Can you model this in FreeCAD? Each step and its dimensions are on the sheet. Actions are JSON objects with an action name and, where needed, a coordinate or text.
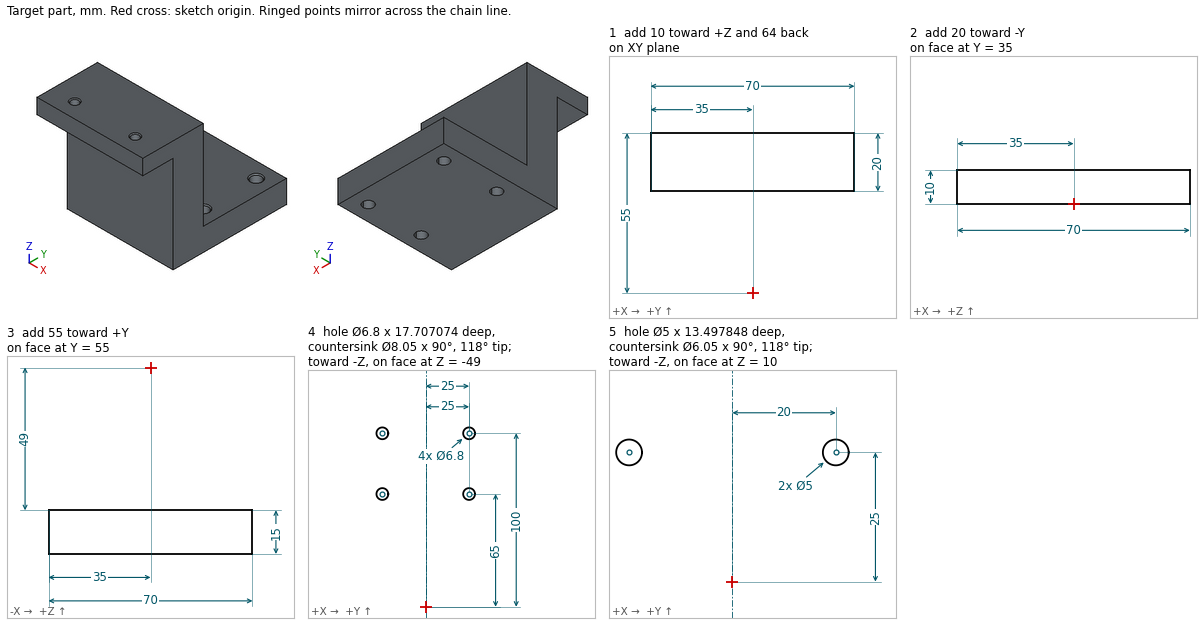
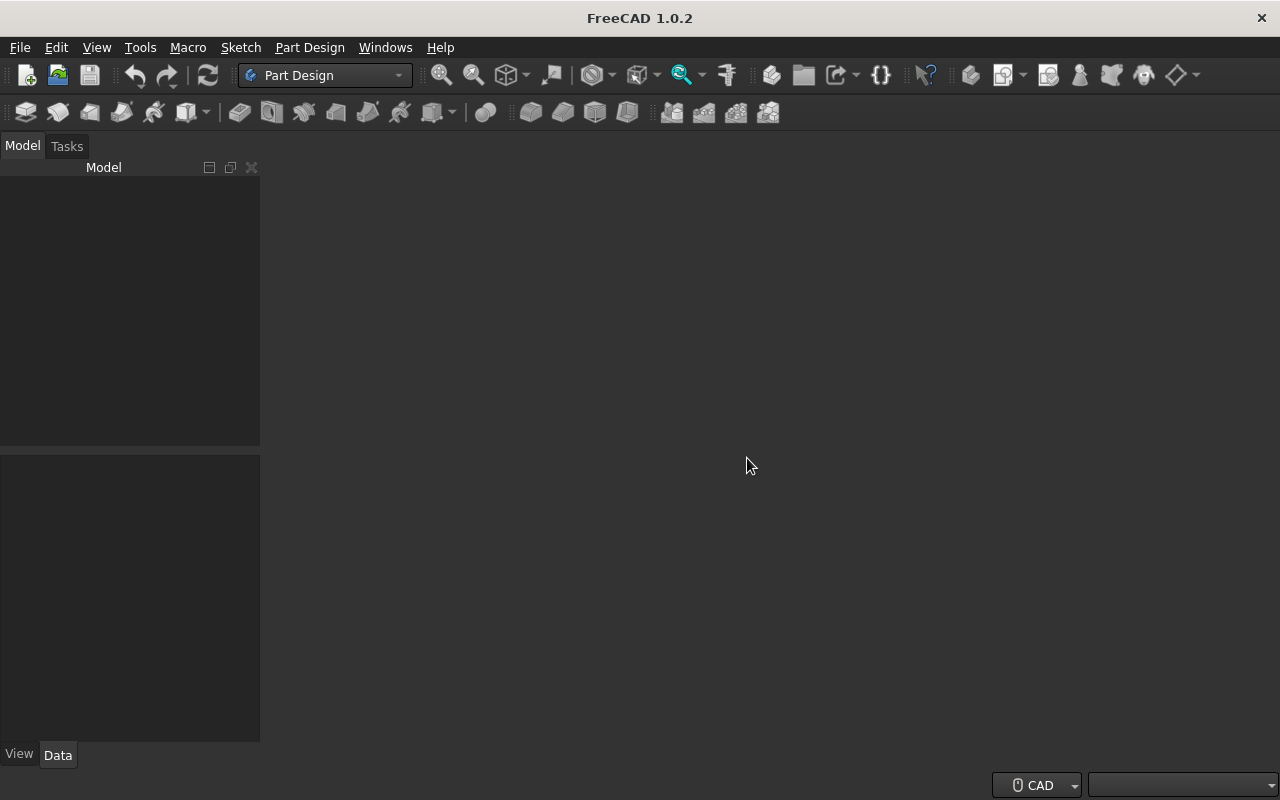
{"action": "left_click", "coordinate": [26, 76]}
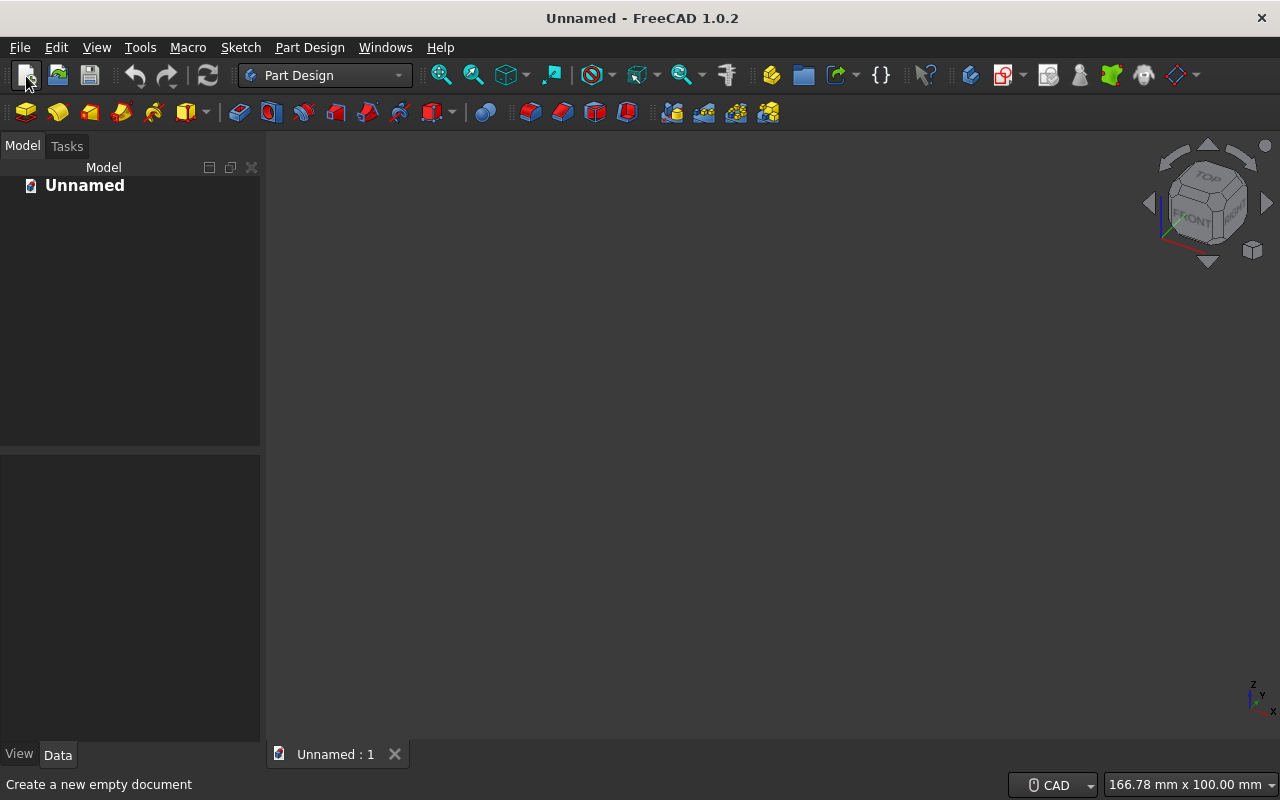
{"action": "left_click", "coordinate": [1004, 76]}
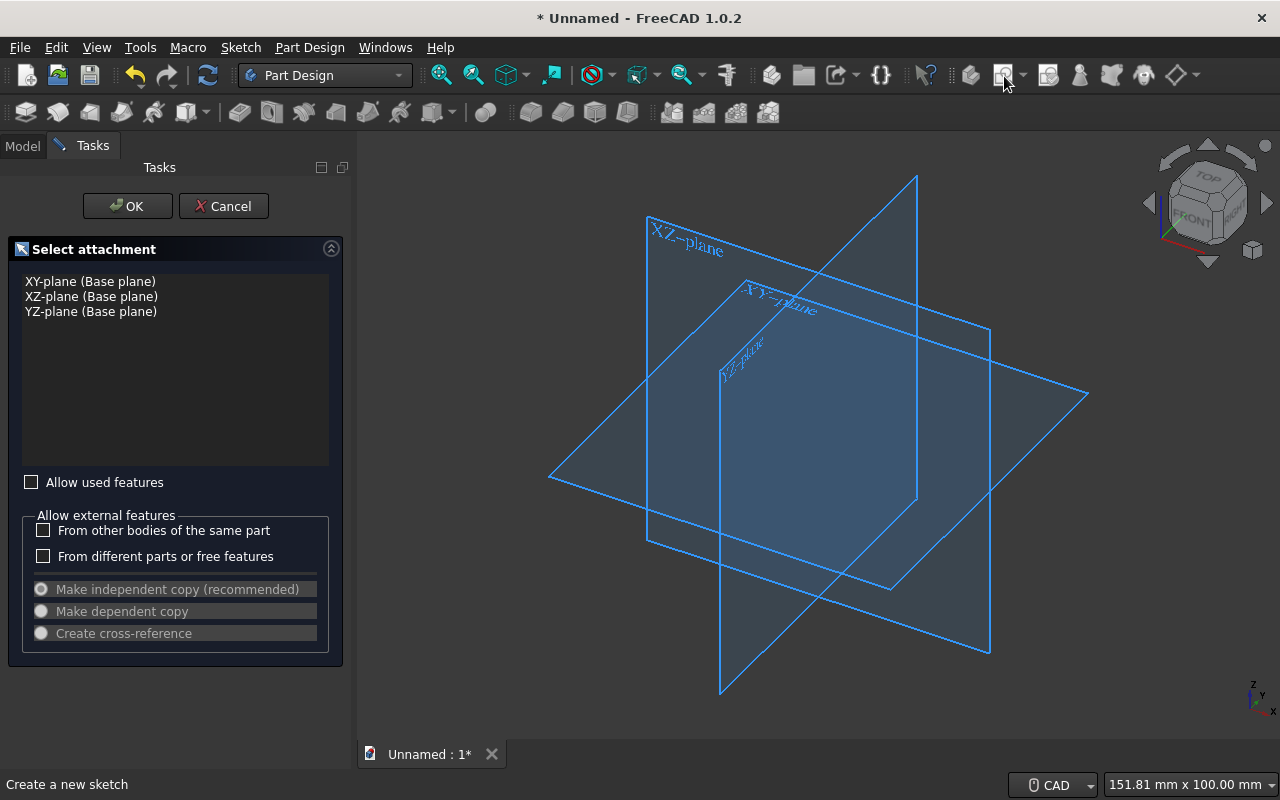
{"action": "left_click", "coordinate": [82, 282]}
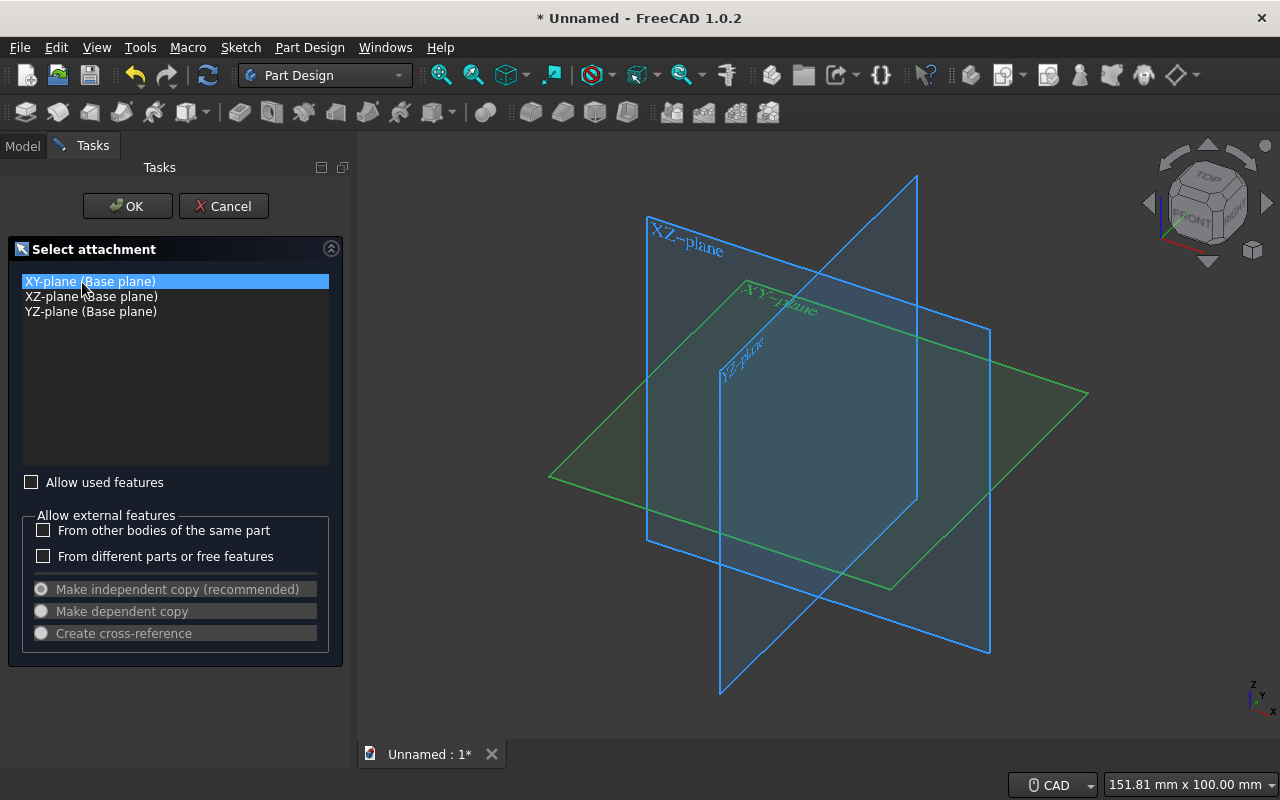
{"action": "left_click", "coordinate": [128, 206]}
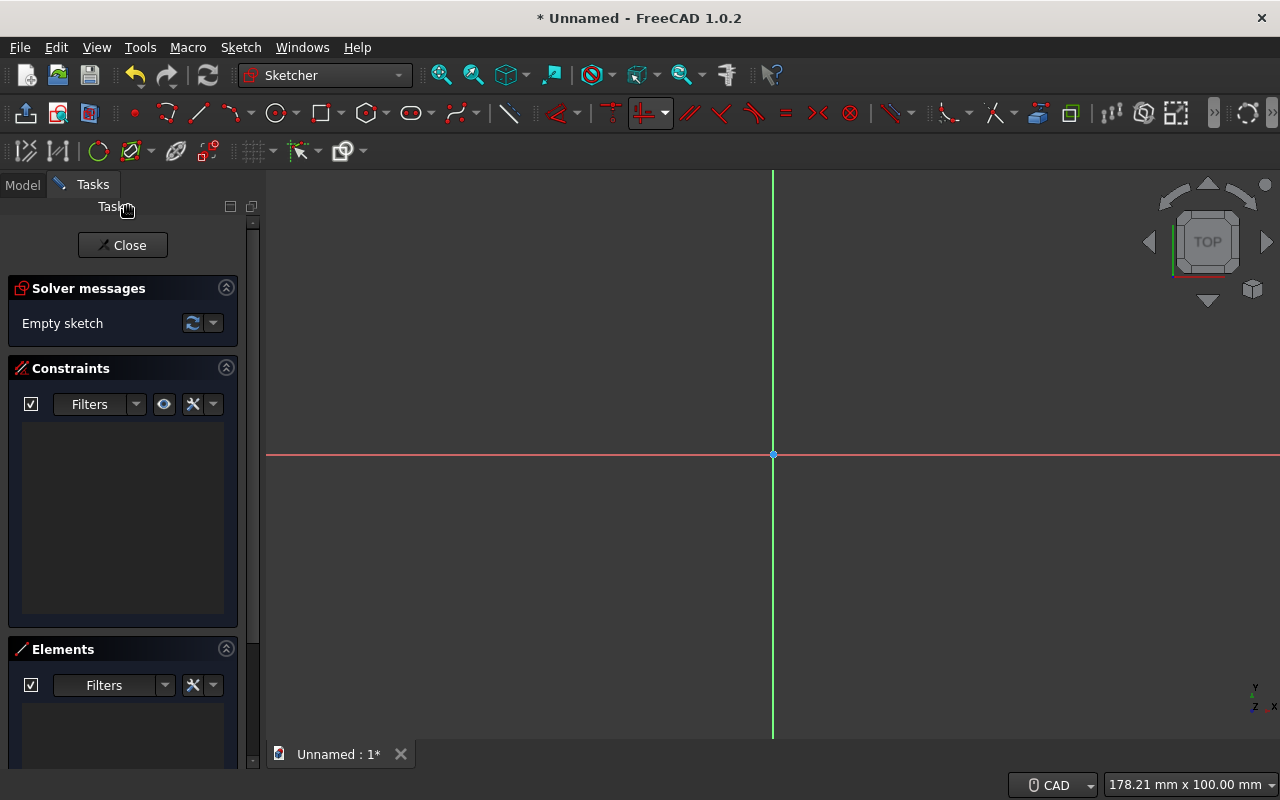
{"action": "scroll", "coordinate": [395, 711], "scroll_direction": "down", "scroll_amount": 1}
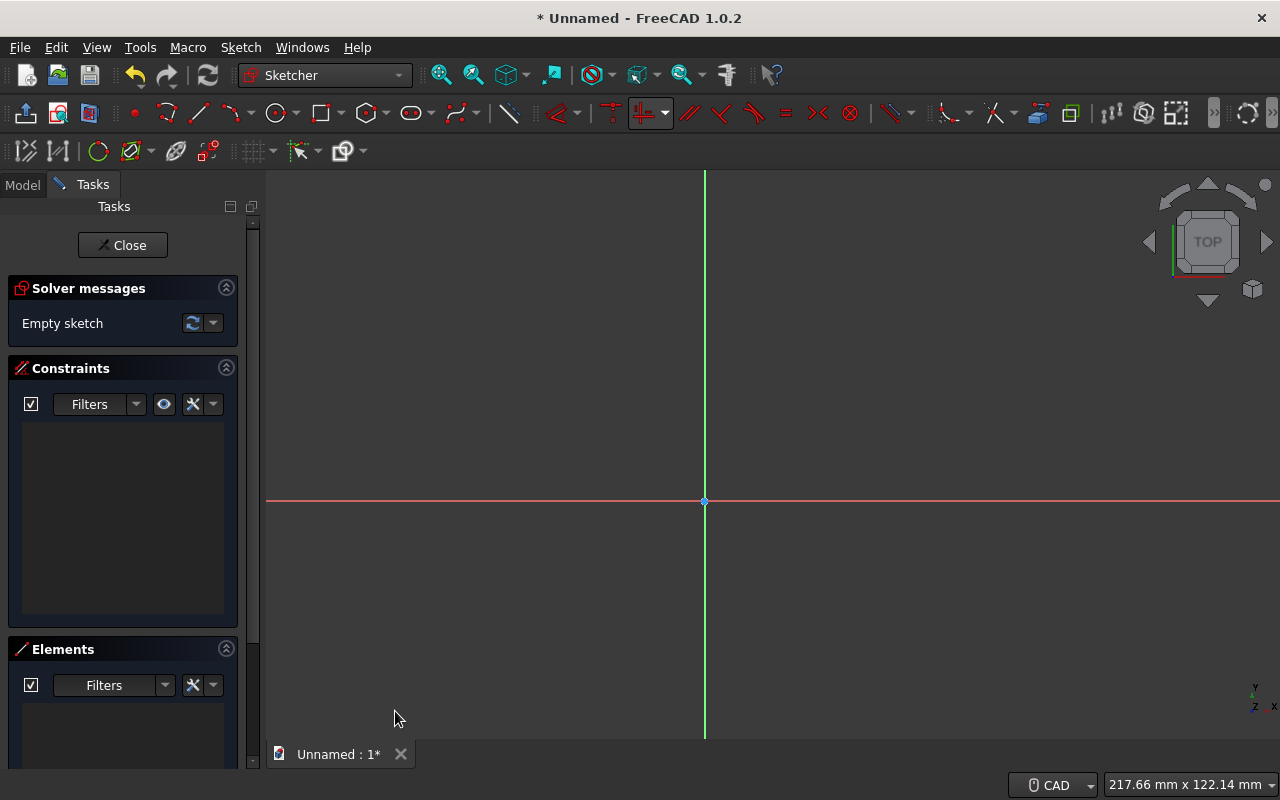
{"action": "scroll", "coordinate": [705, 207], "scroll_direction": "up", "scroll_amount": 2}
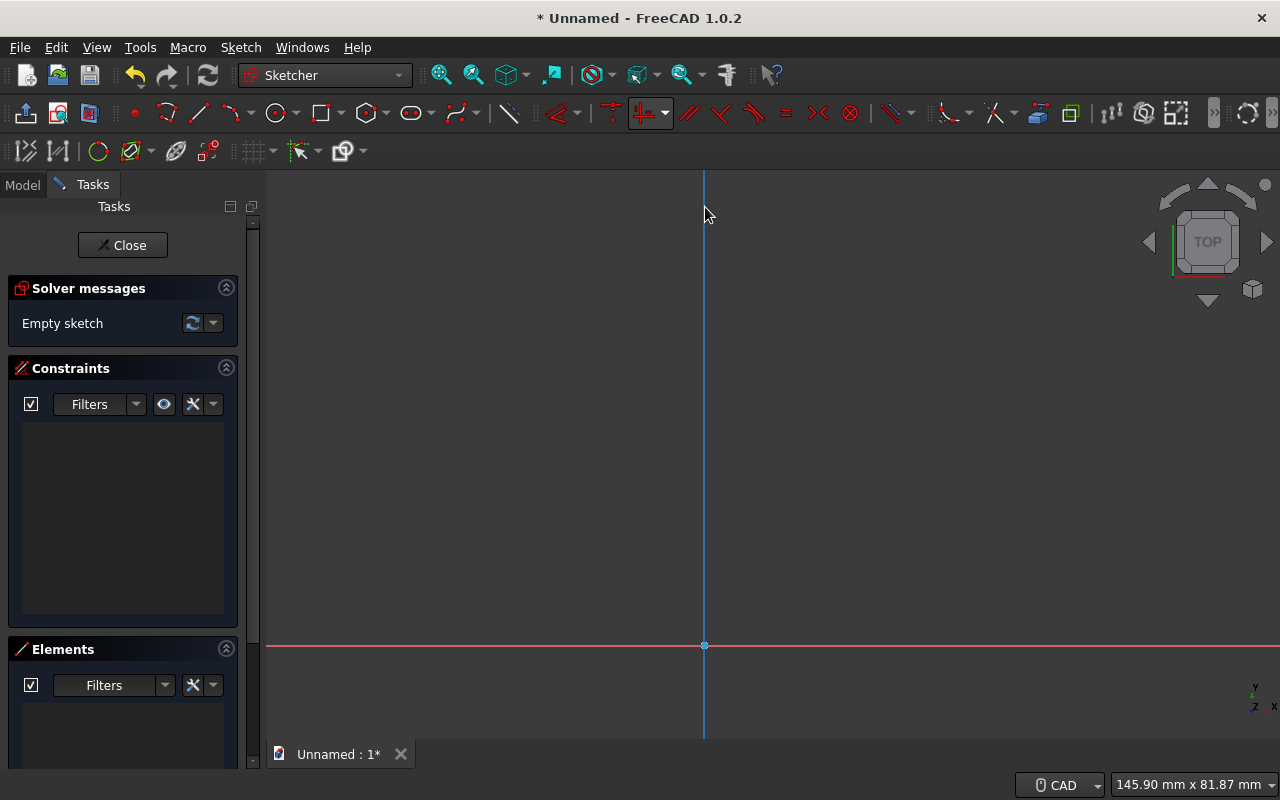
{"action": "key", "text": "g r"}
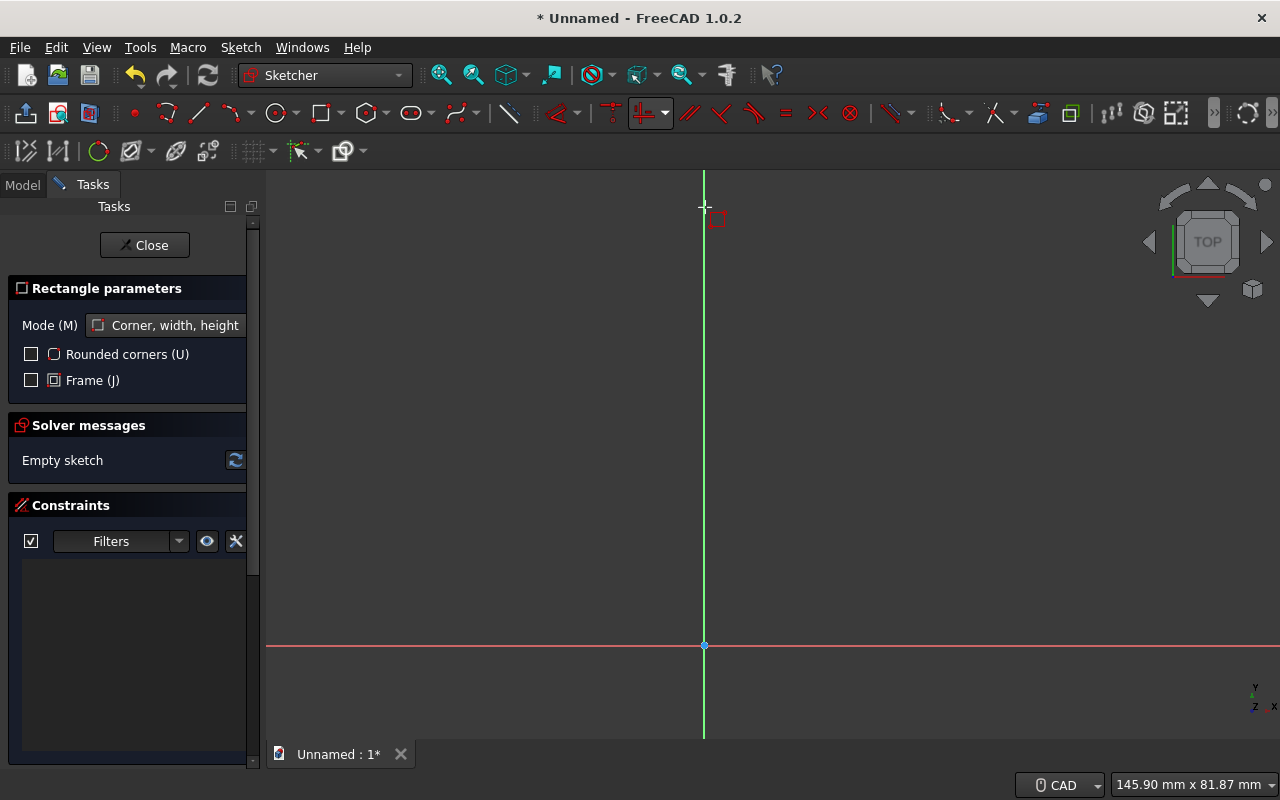
{"action": "left_click", "coordinate": [461, 264]}
{"action": "mouse_move", "coordinate": [947, 403]}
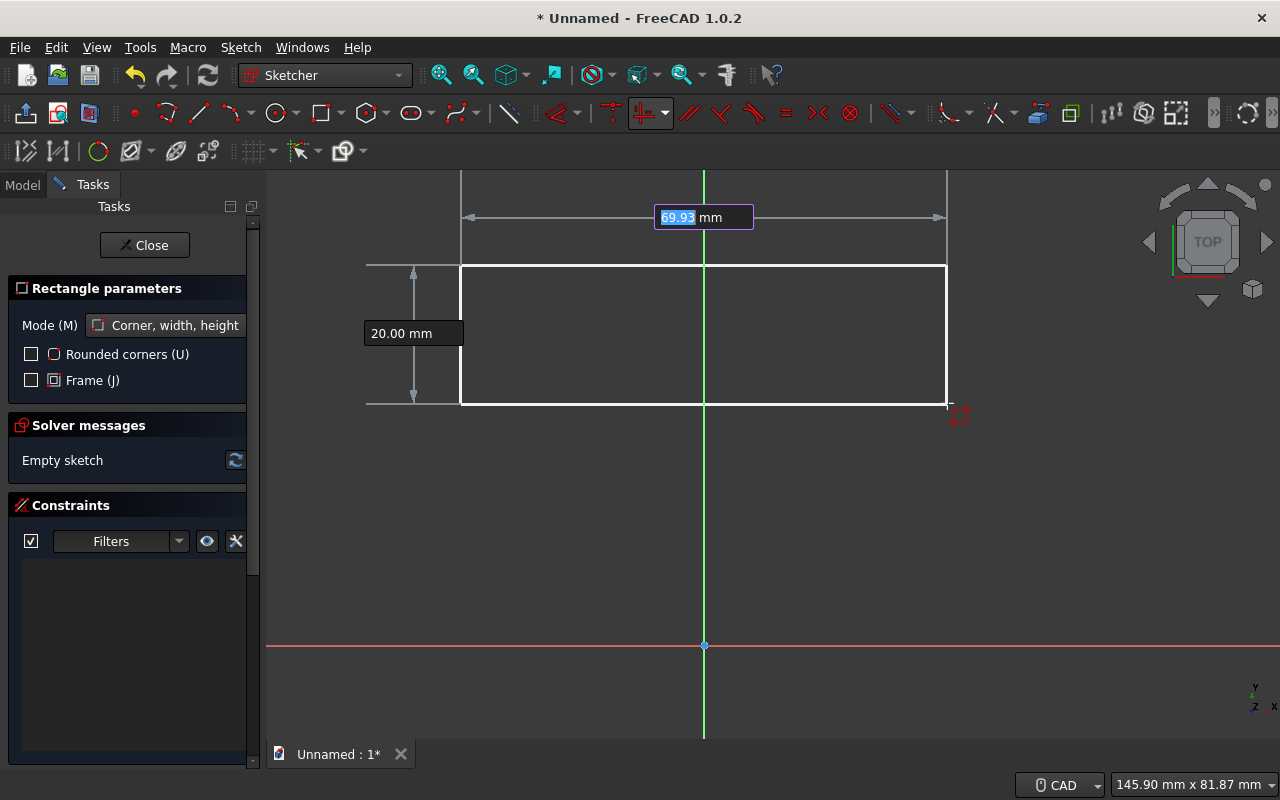
{"action": "type", "text": "70"}
{"action": "key", "text": "Tab"}
{"action": "type", "text": "20"}
{"action": "key", "text": "Return"}
{"action": "key", "text": "Escape"}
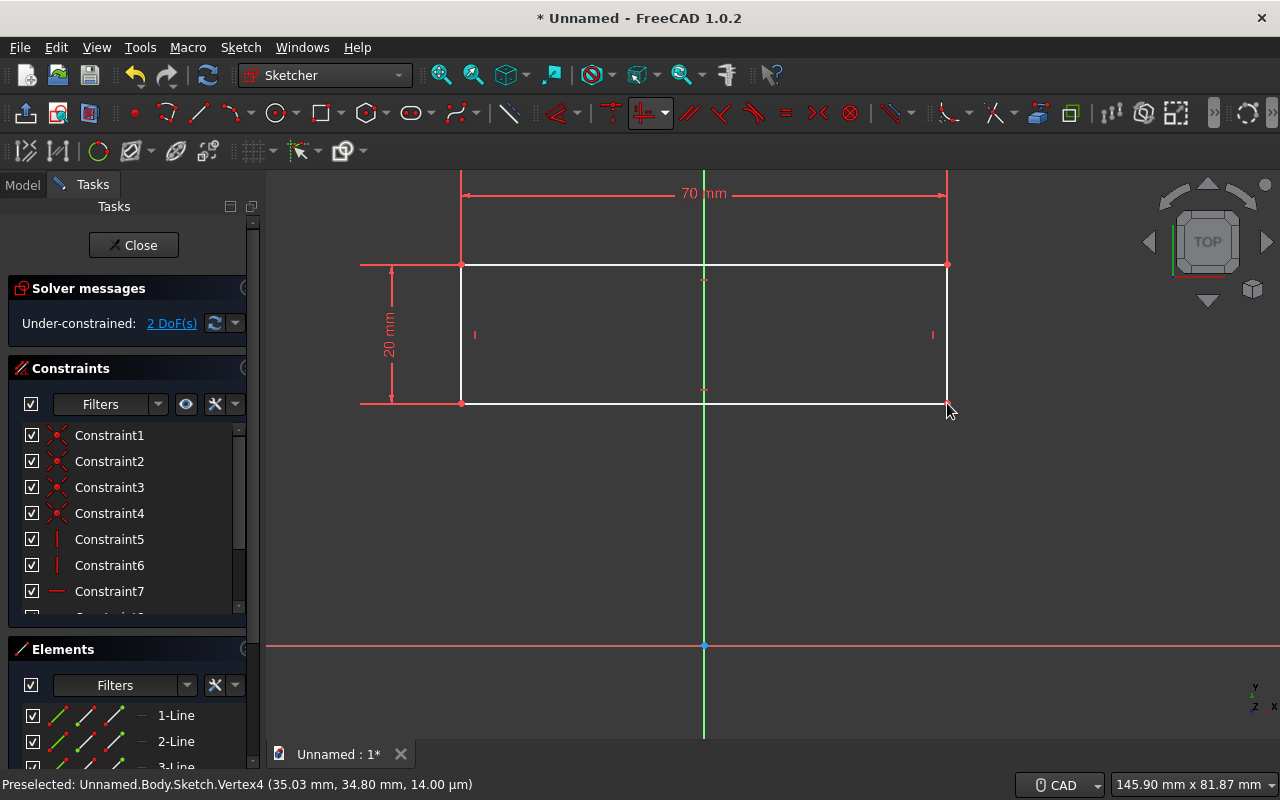
{"action": "left_click", "coordinate": [461, 265]}